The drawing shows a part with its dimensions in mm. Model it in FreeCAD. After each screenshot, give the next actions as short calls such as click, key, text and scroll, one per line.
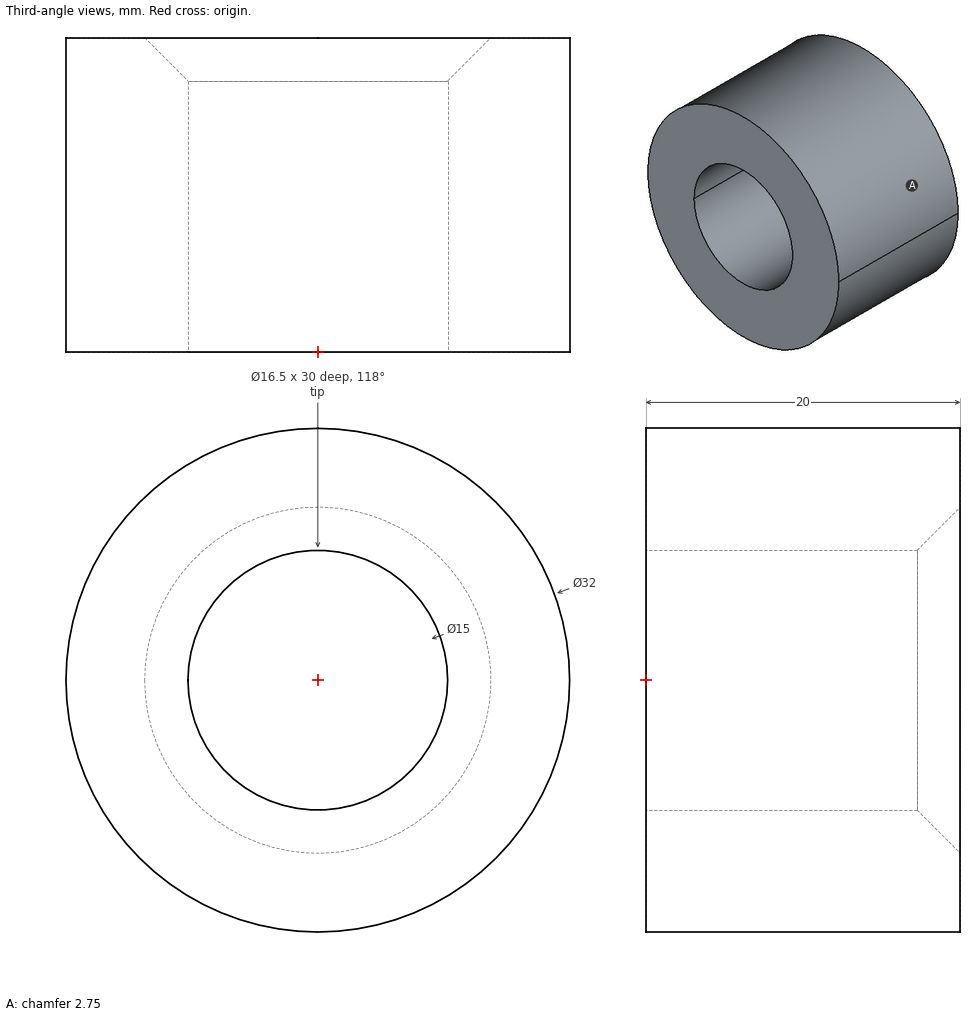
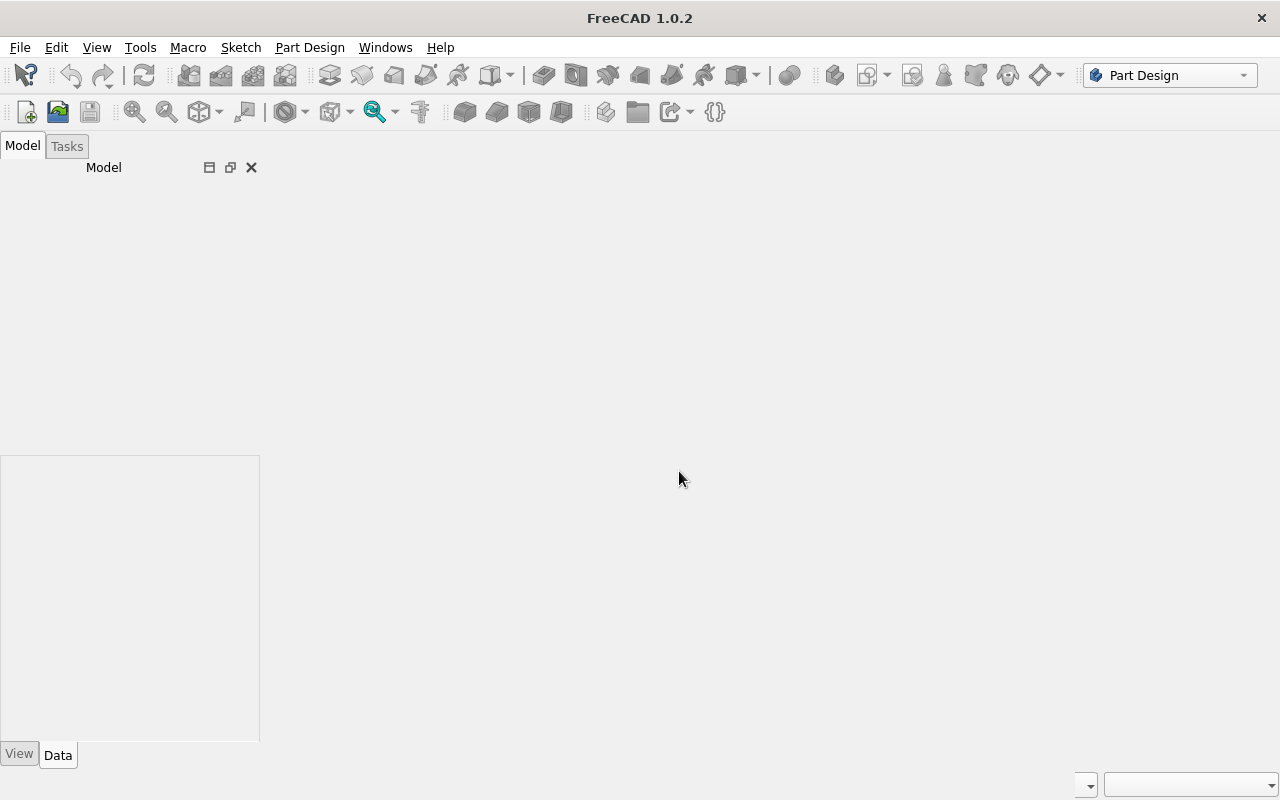
click(26, 112)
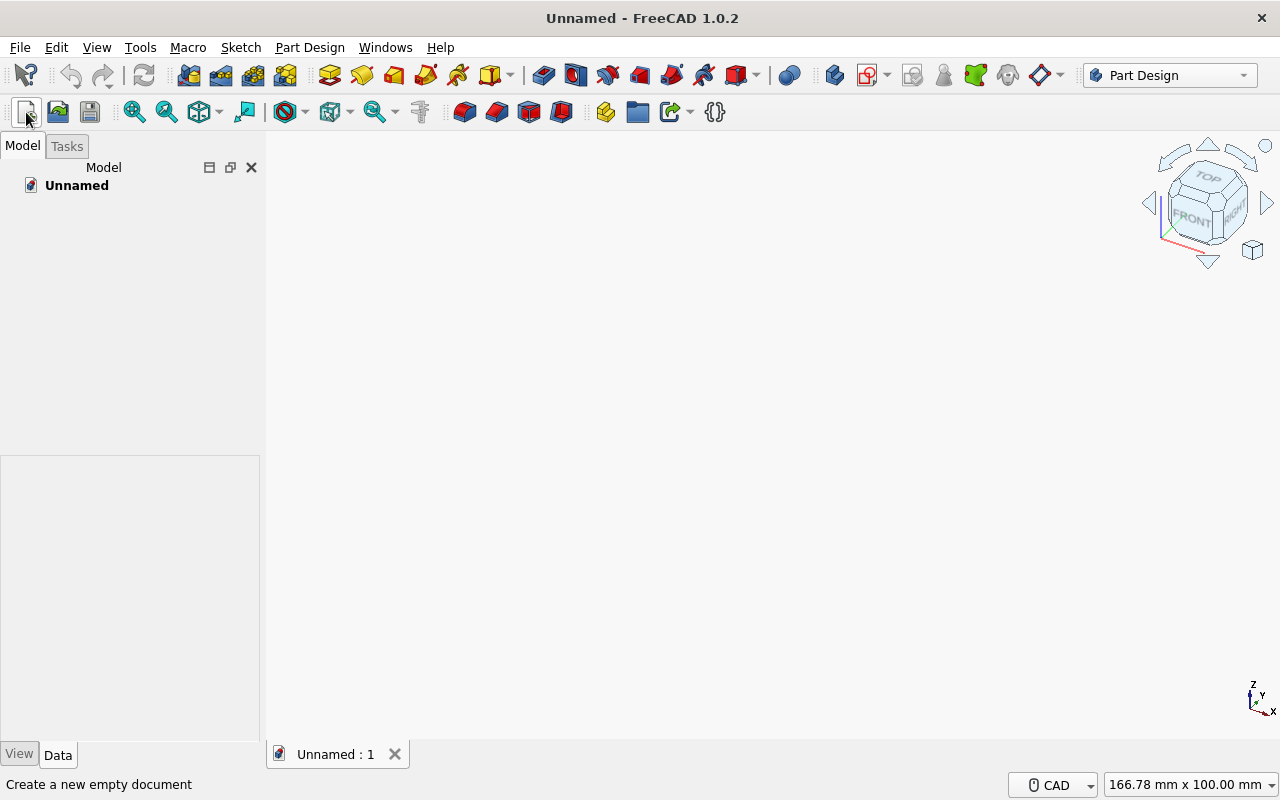
click(868, 76)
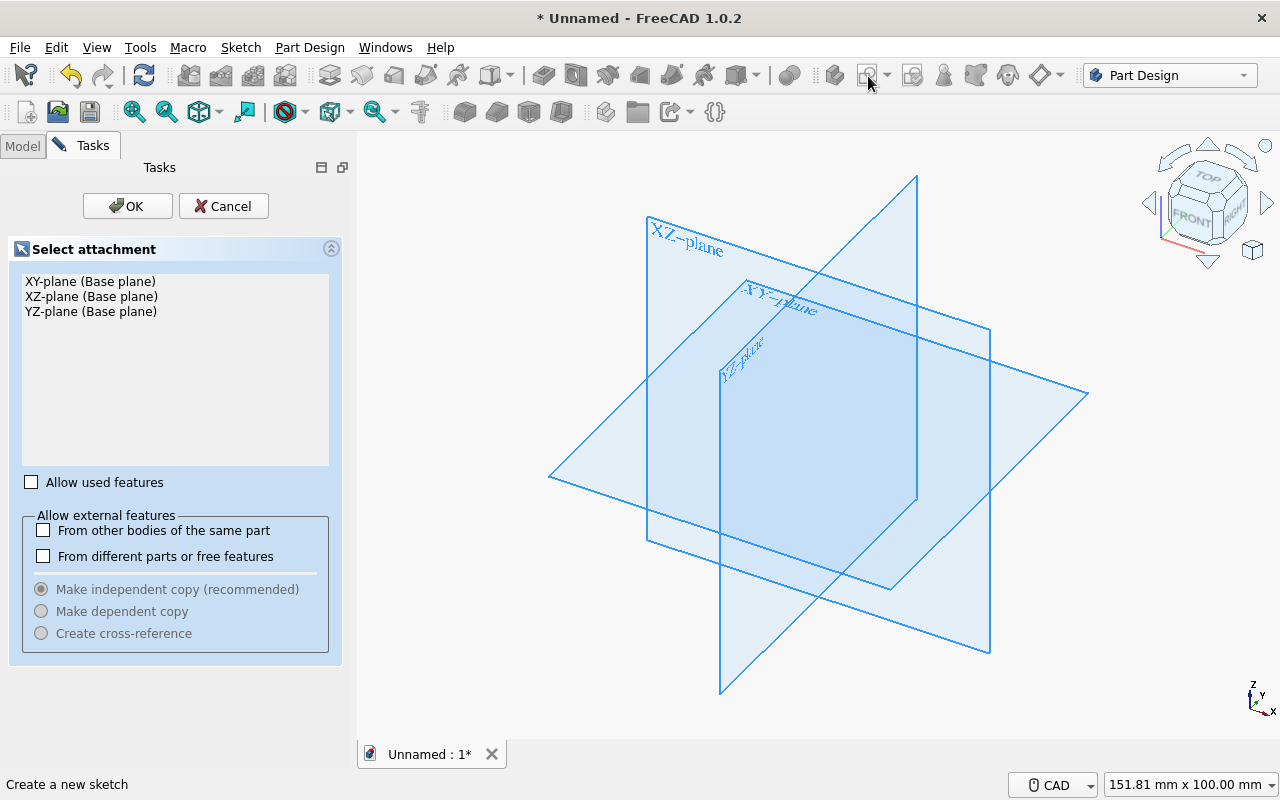
click(82, 296)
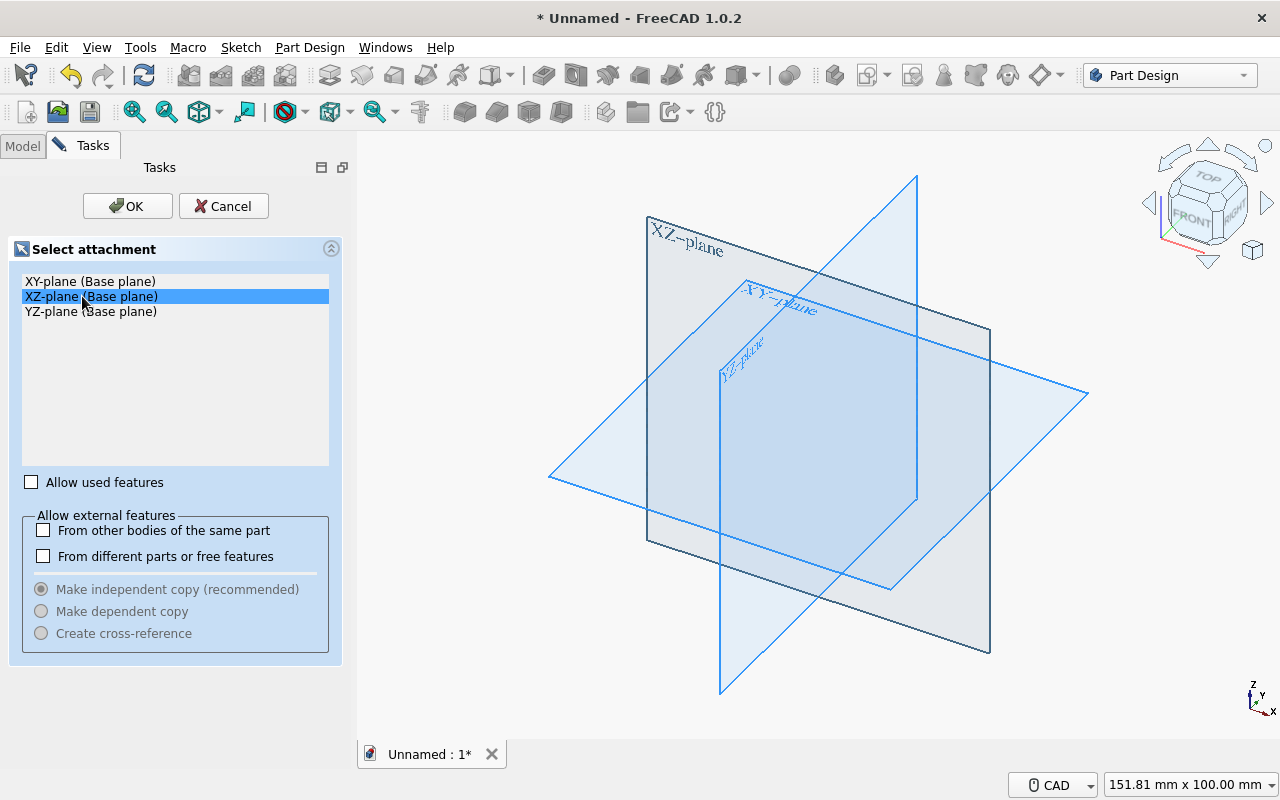
click(128, 206)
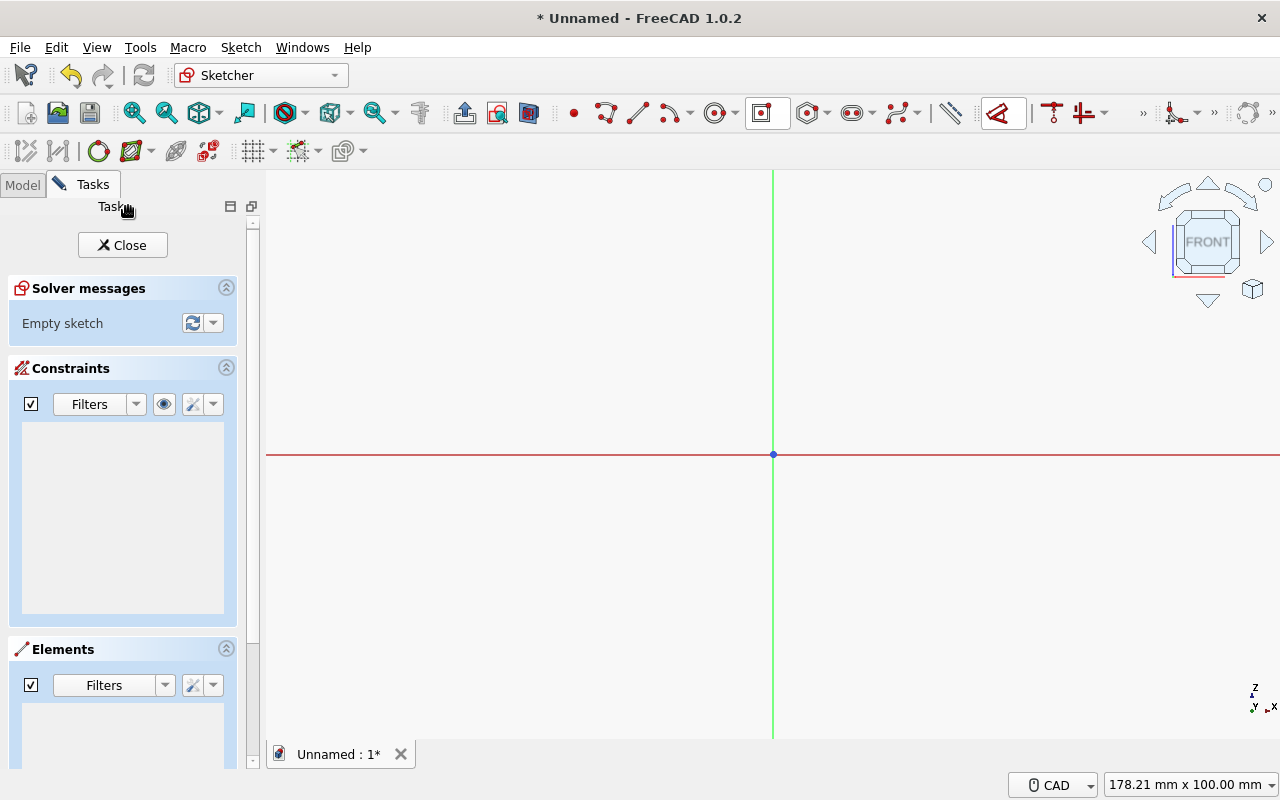
scroll(856, 454, up, 3)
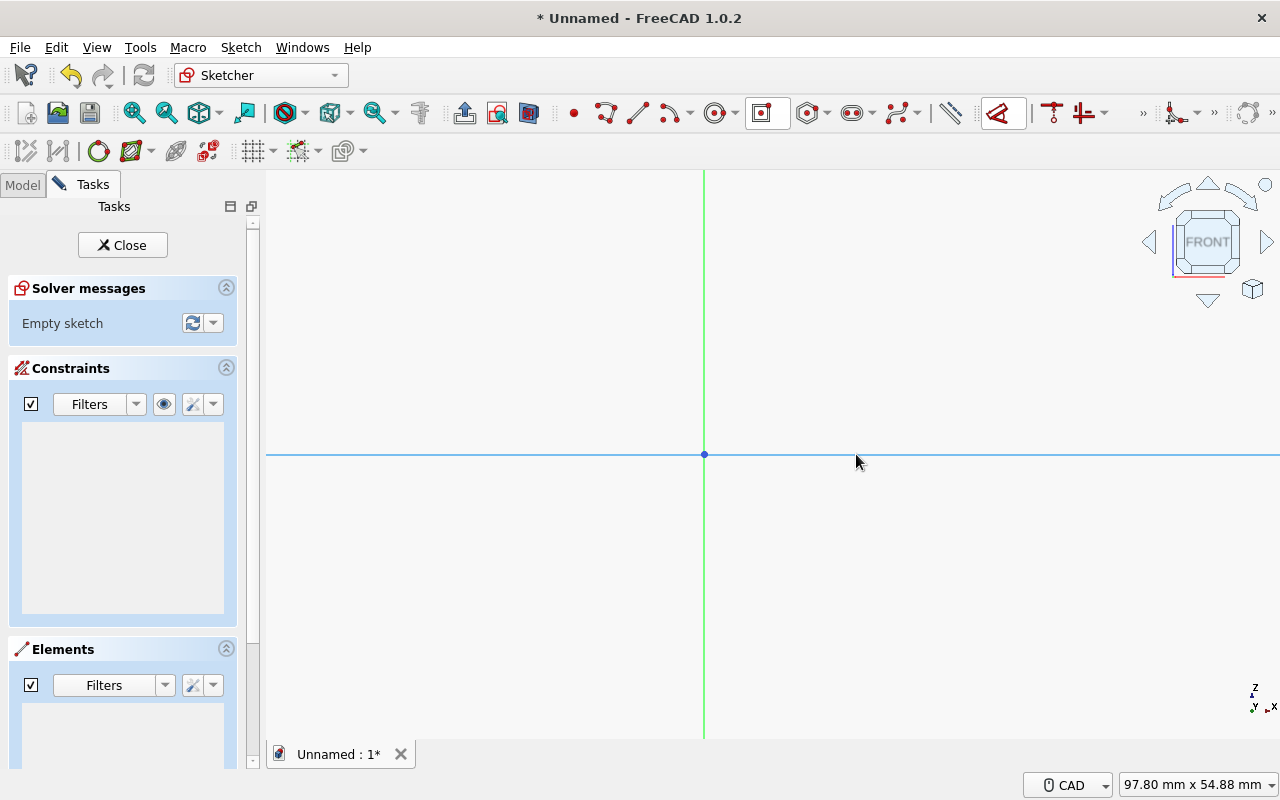
click(716, 114)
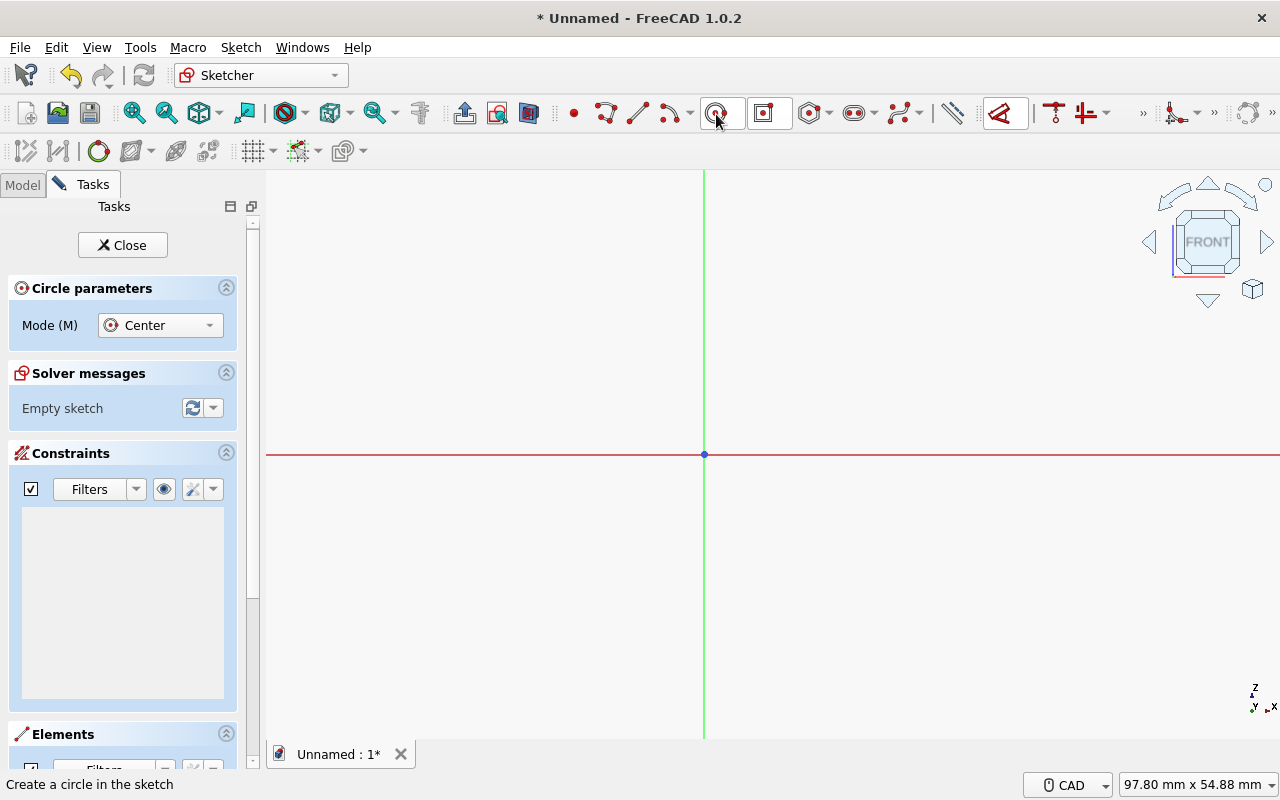
click(704, 454)
move(822, 337)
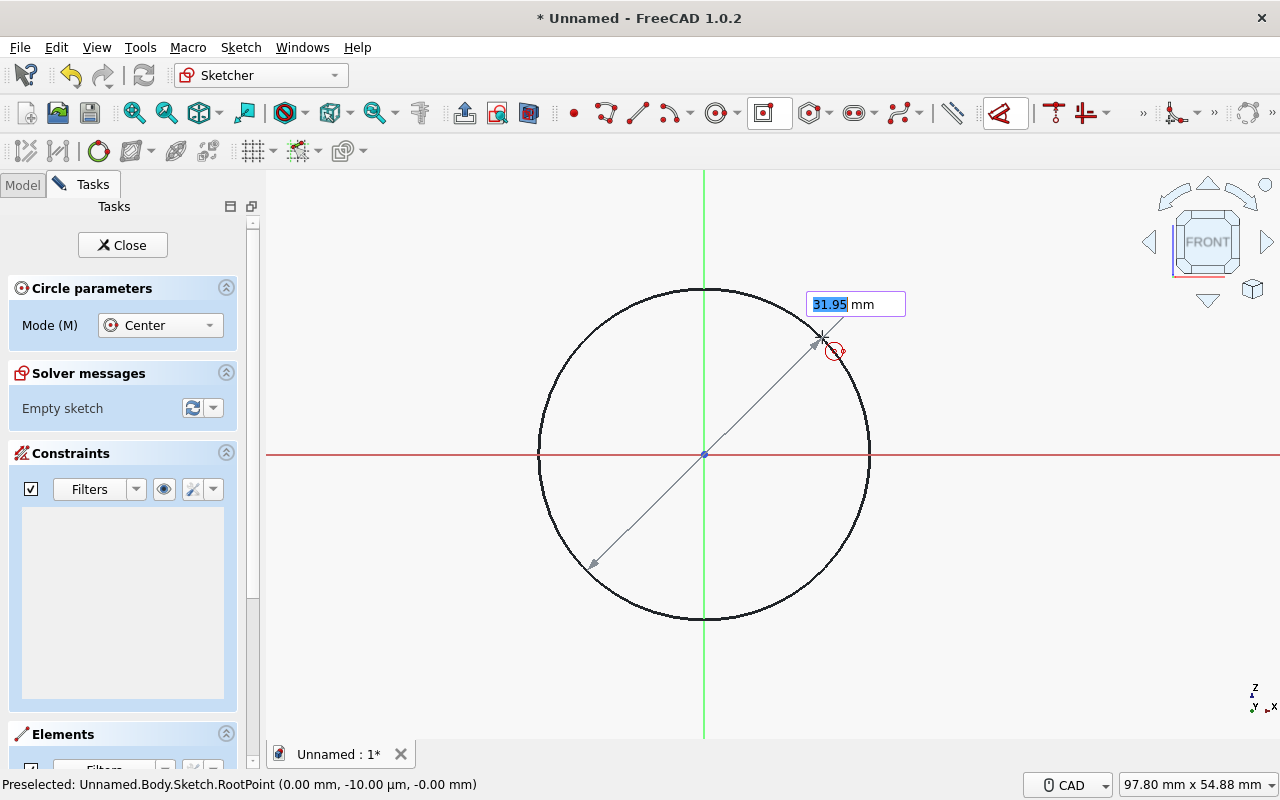
text(32)
key(Return)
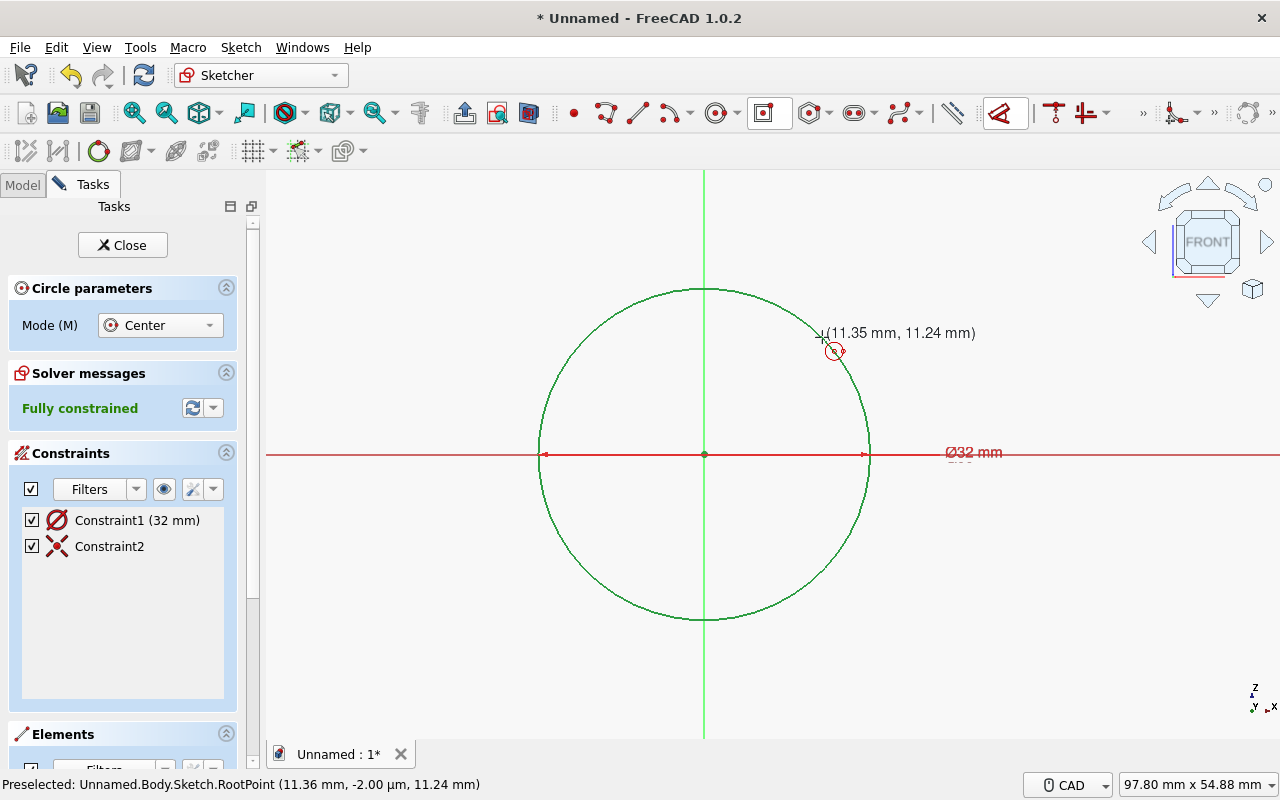
click(704, 454)
move(759, 400)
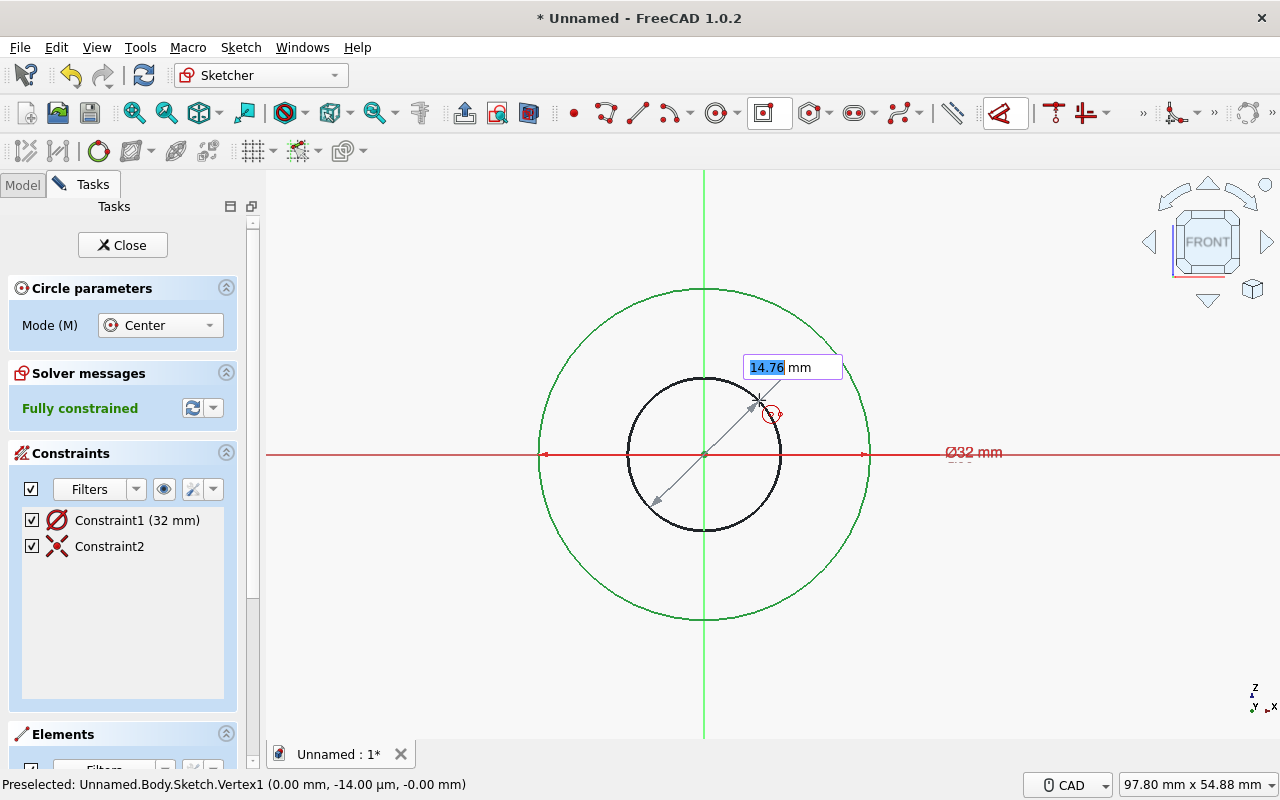
text(15)
key(Return)
key(Escape)